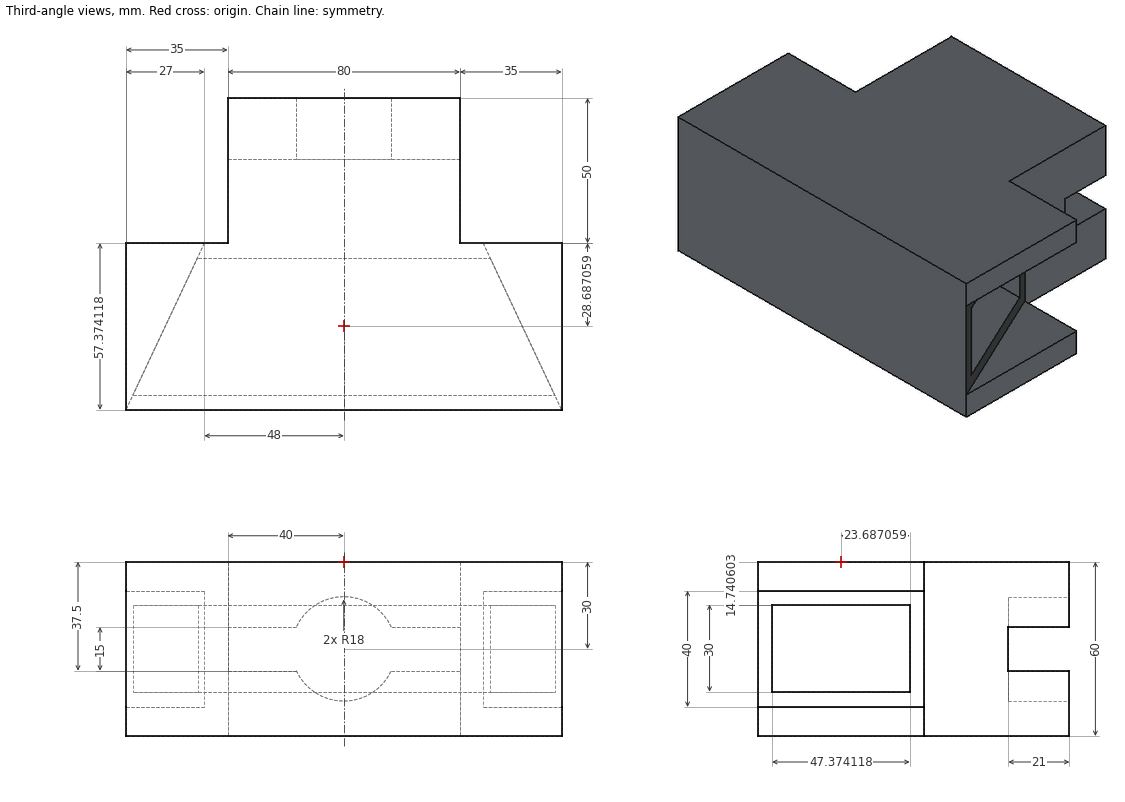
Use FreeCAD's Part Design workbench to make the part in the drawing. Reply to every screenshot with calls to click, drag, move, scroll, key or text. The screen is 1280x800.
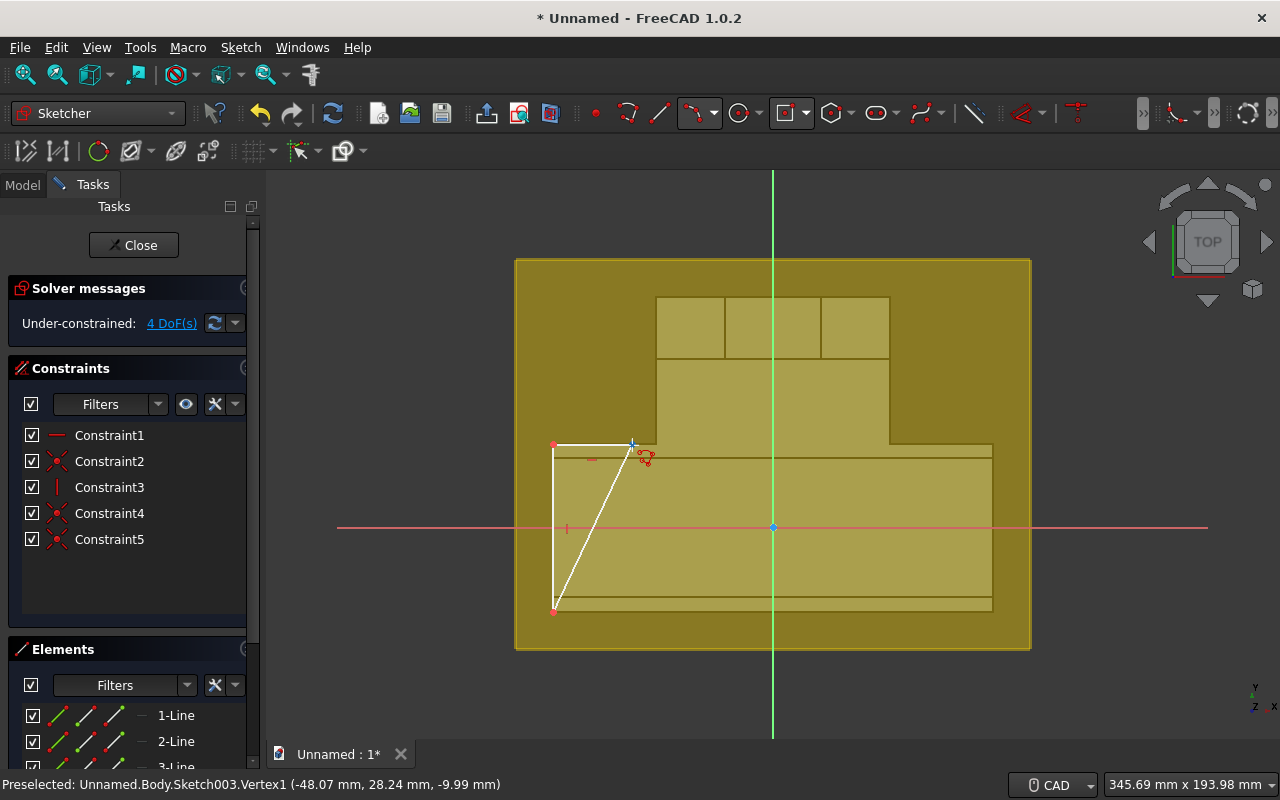
click(914, 444)
click(993, 612)
click(993, 444)
click(914, 445)
key(Escape)
key(Escape)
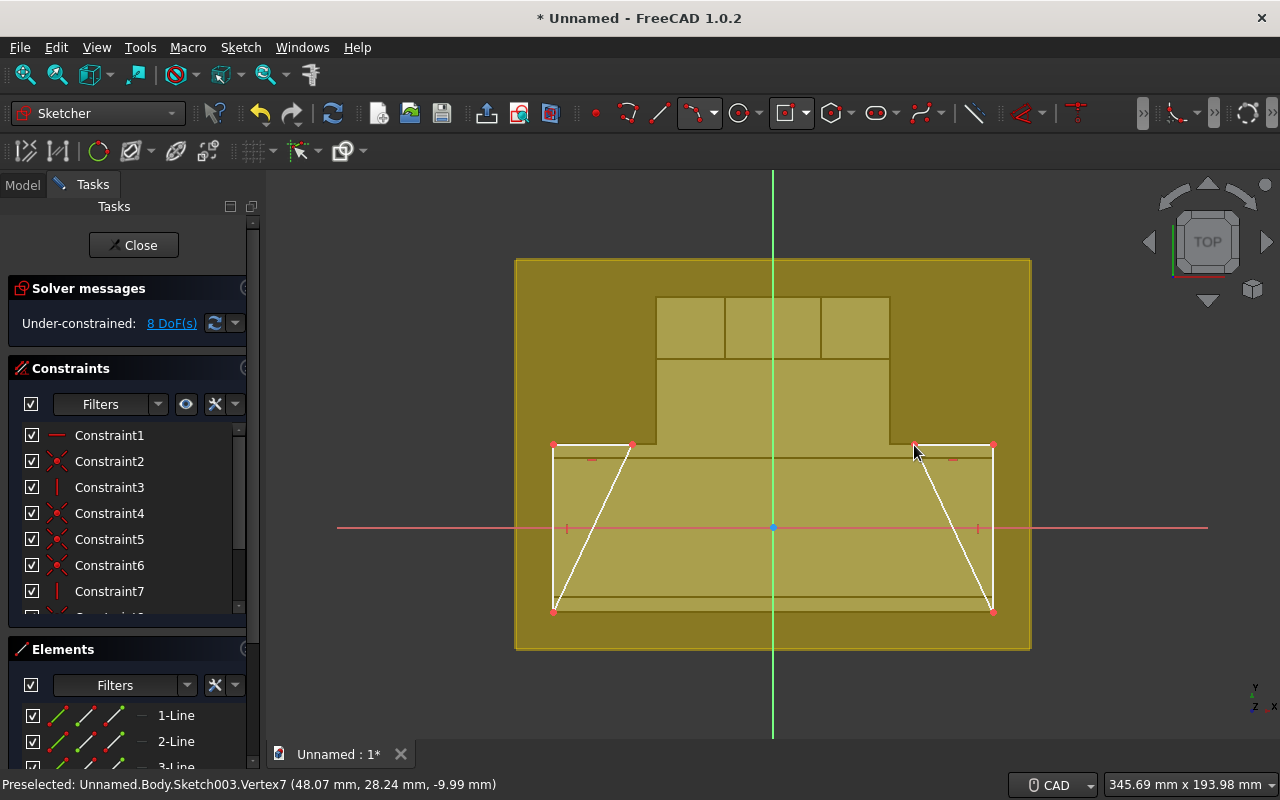
click(632, 445)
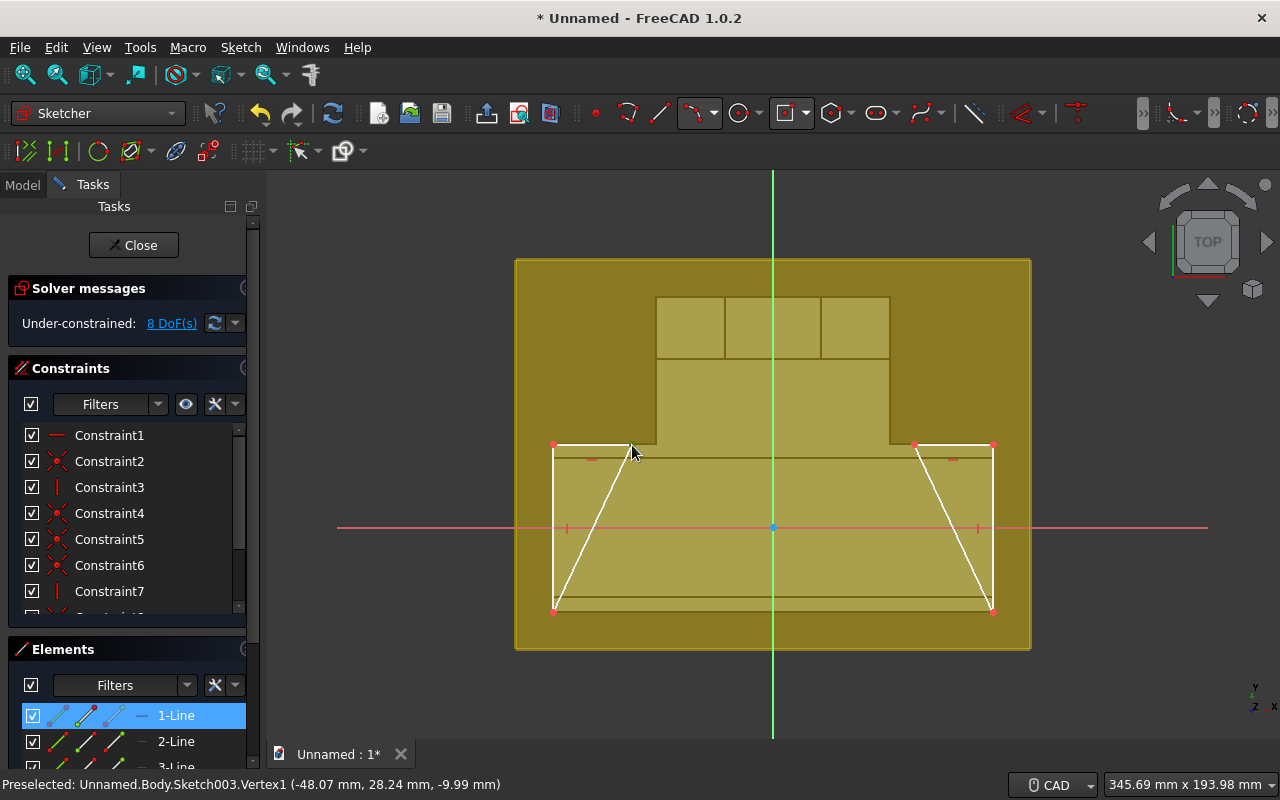
click(914, 445)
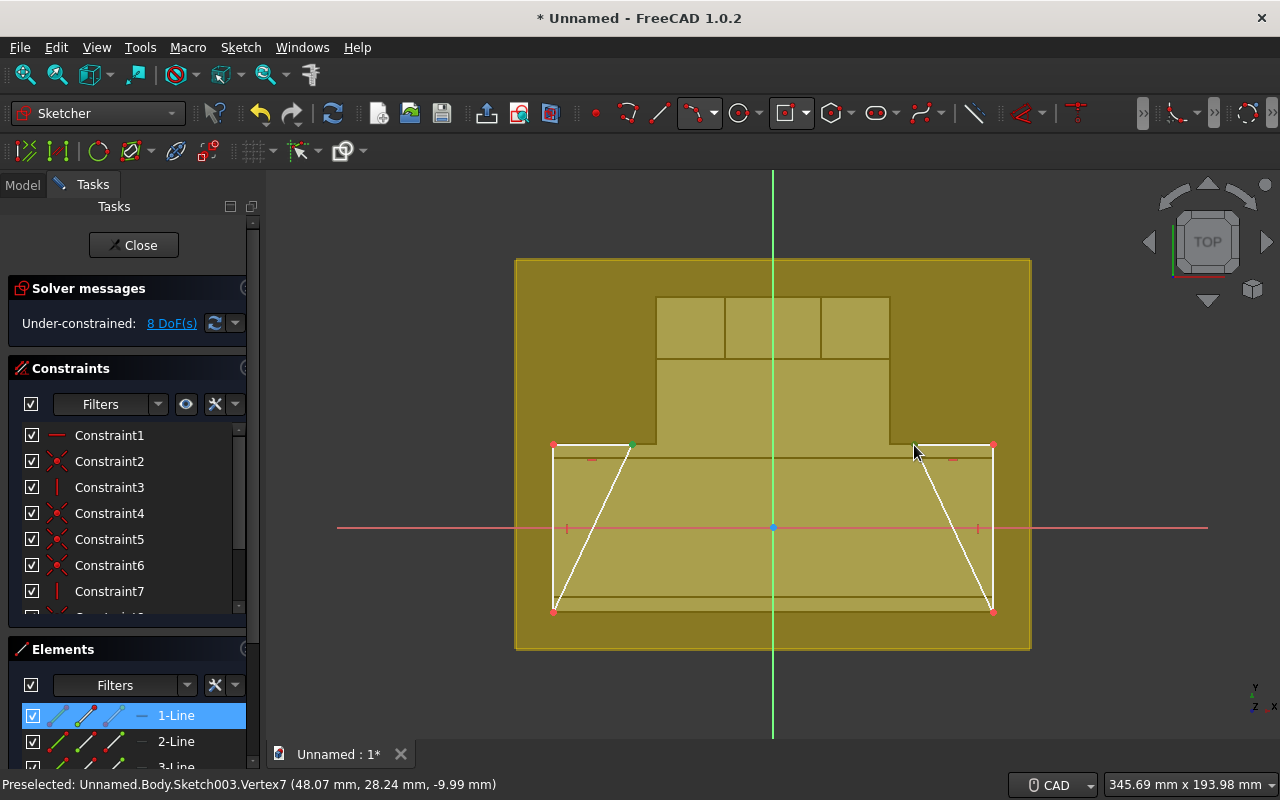
click(773, 674)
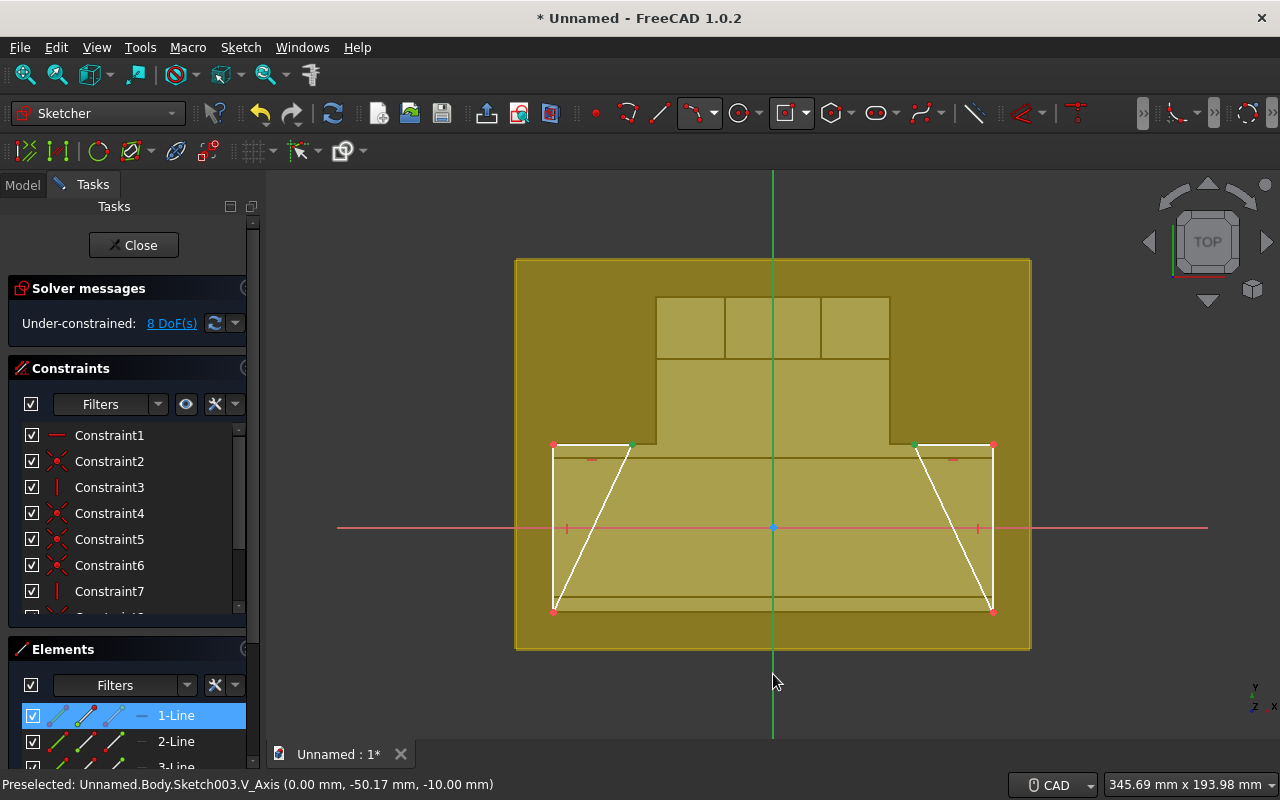
key(s)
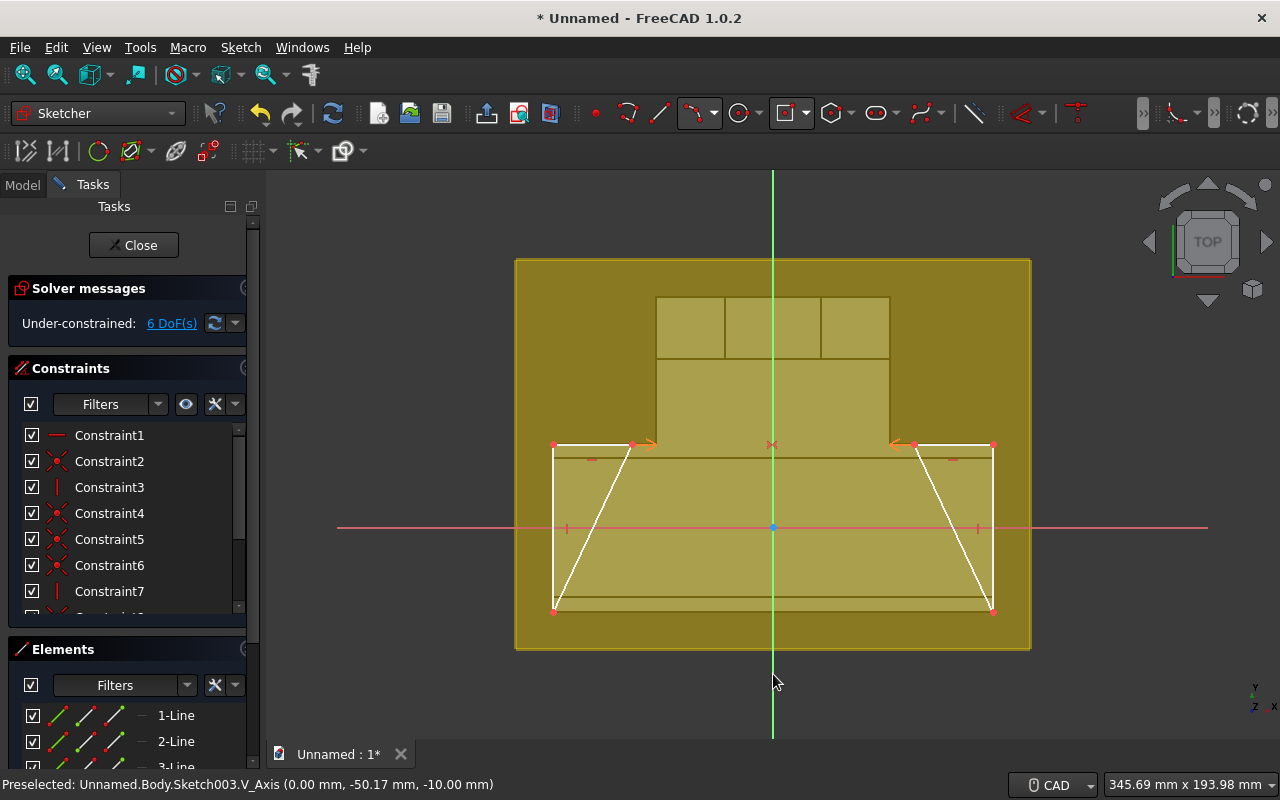
click(553, 613)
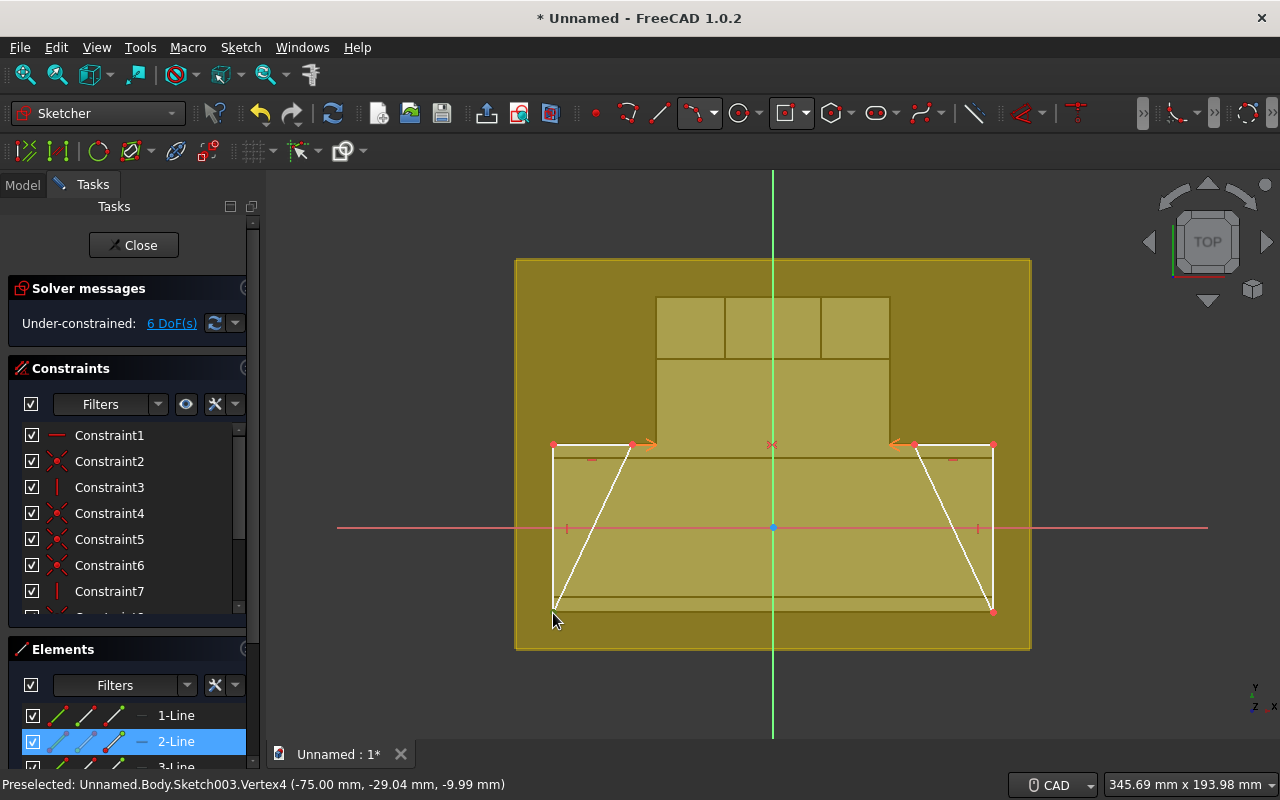
click(993, 613)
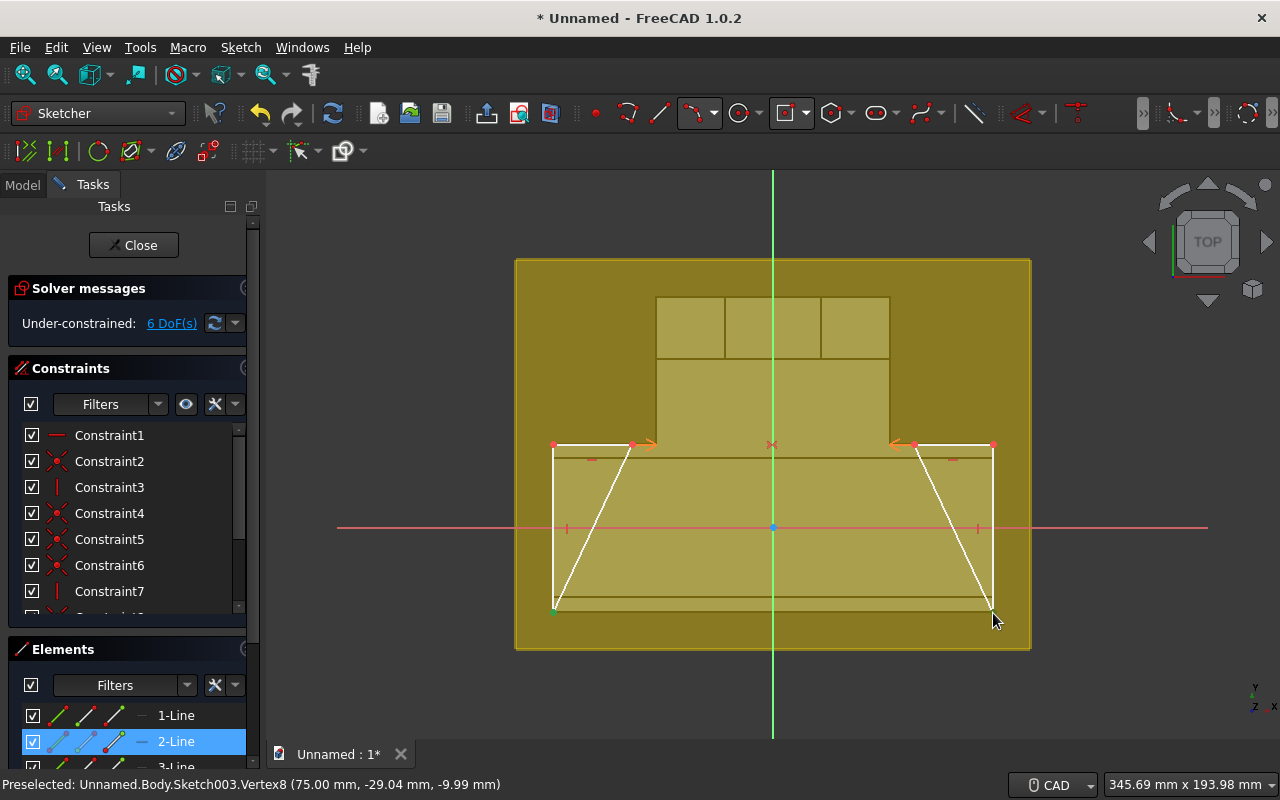
click(773, 674)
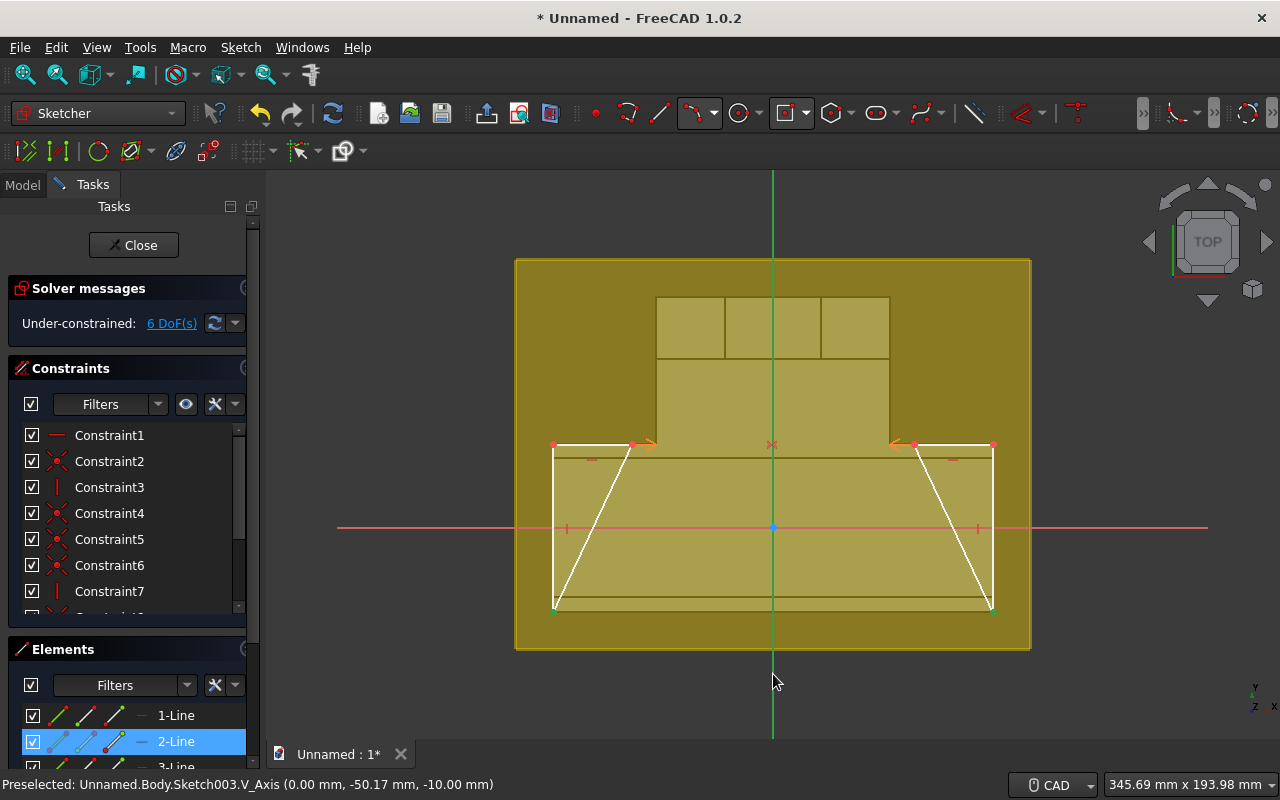
key(s)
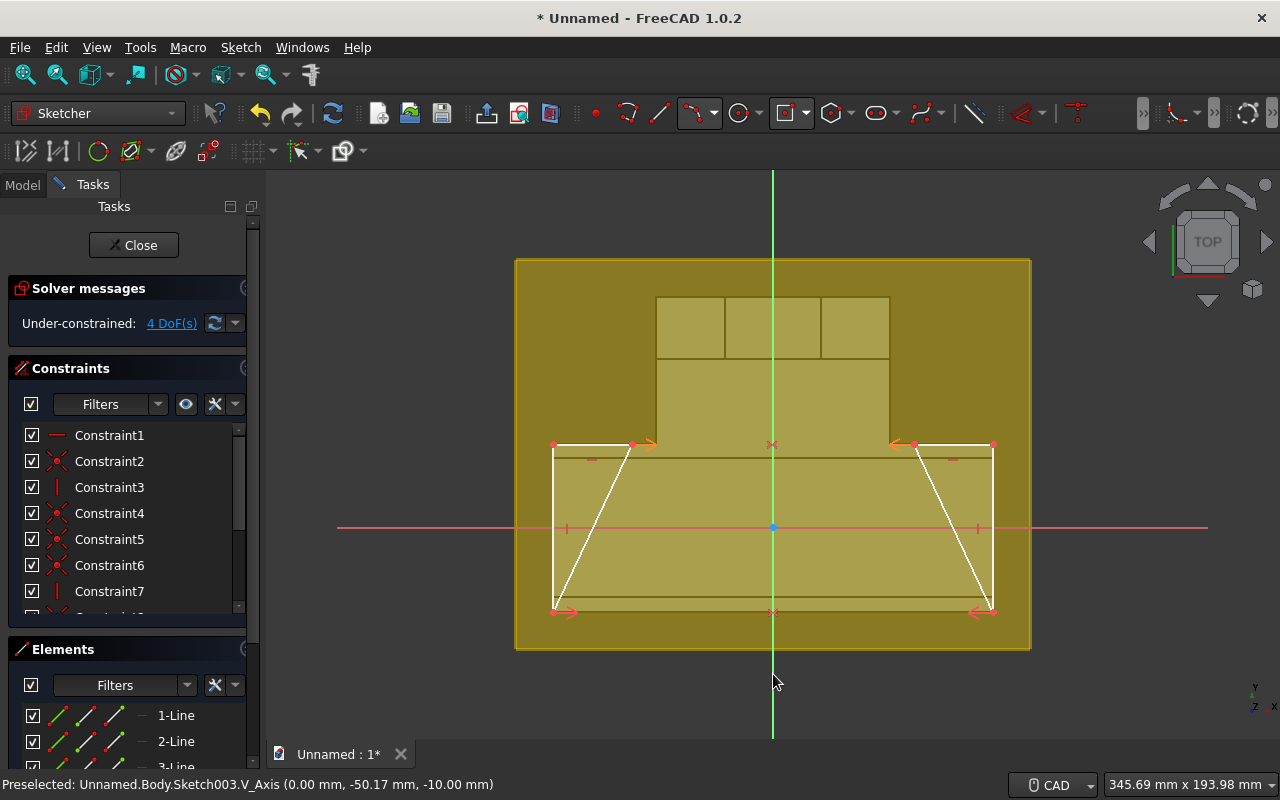
key(d)